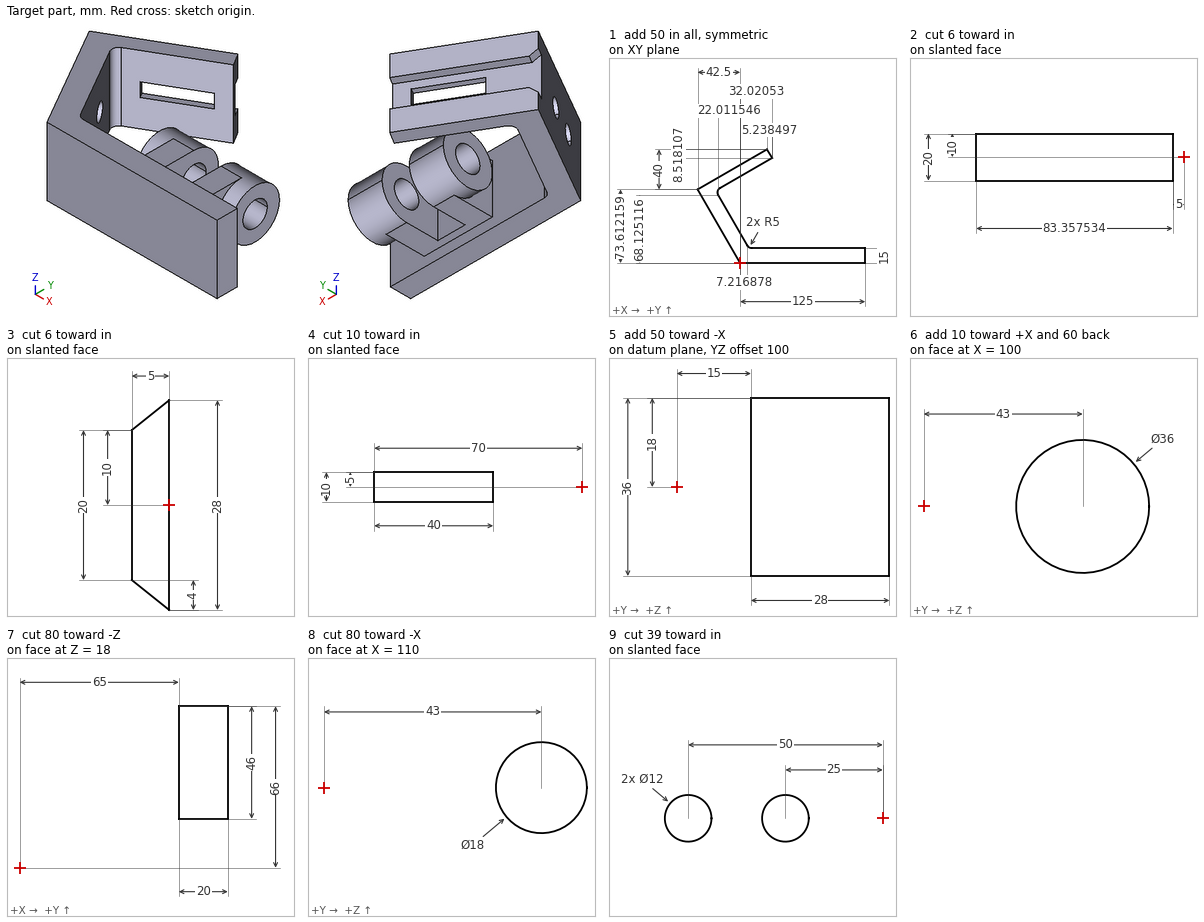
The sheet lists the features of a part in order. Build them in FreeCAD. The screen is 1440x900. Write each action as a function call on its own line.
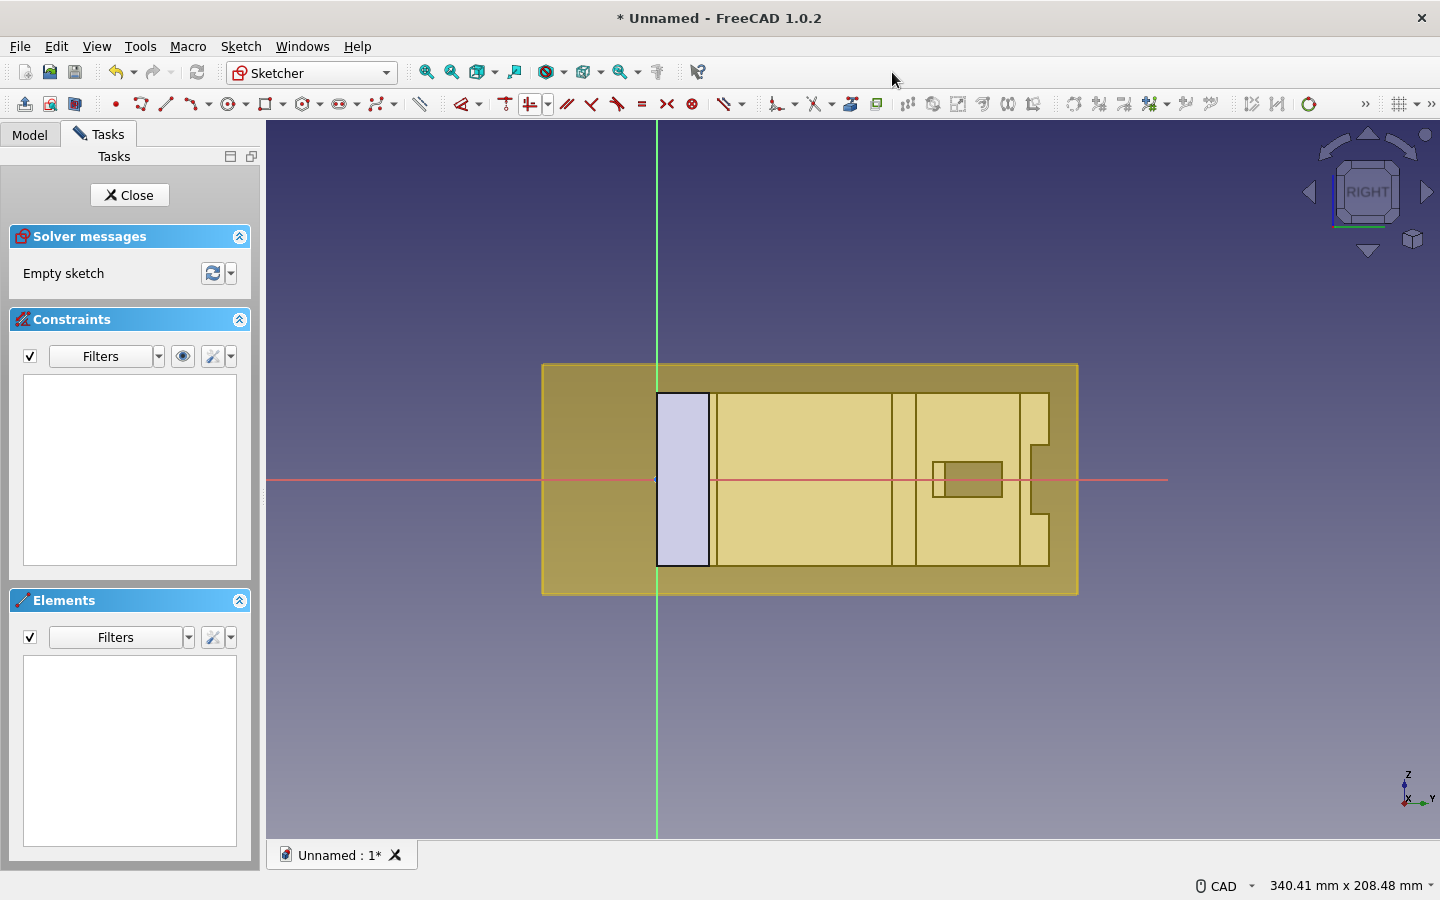
click(75, 104)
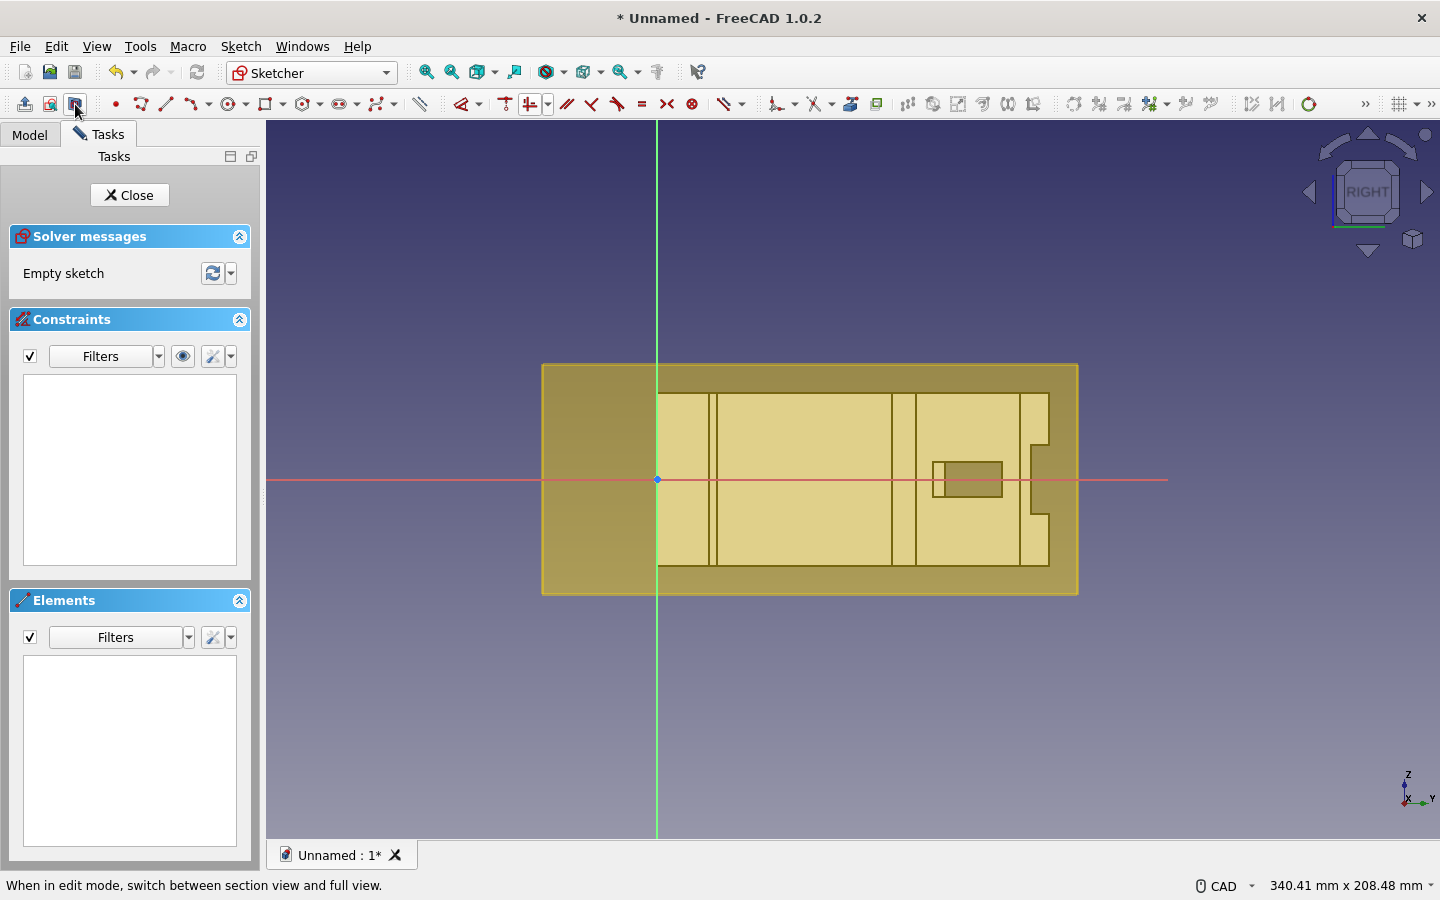
scroll(714, 480, up, 7)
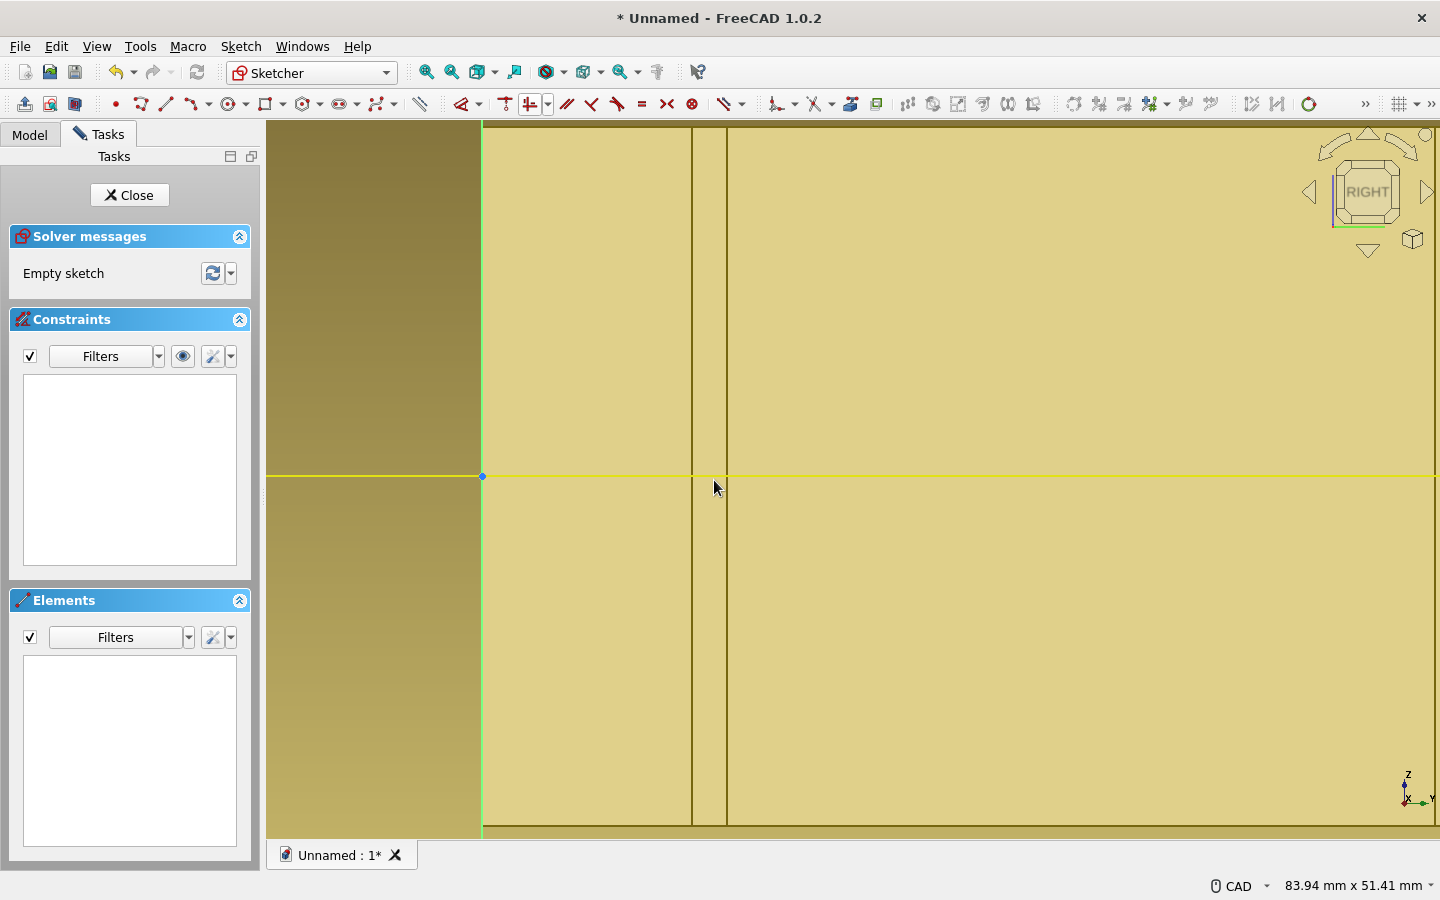
key(g)
key(r)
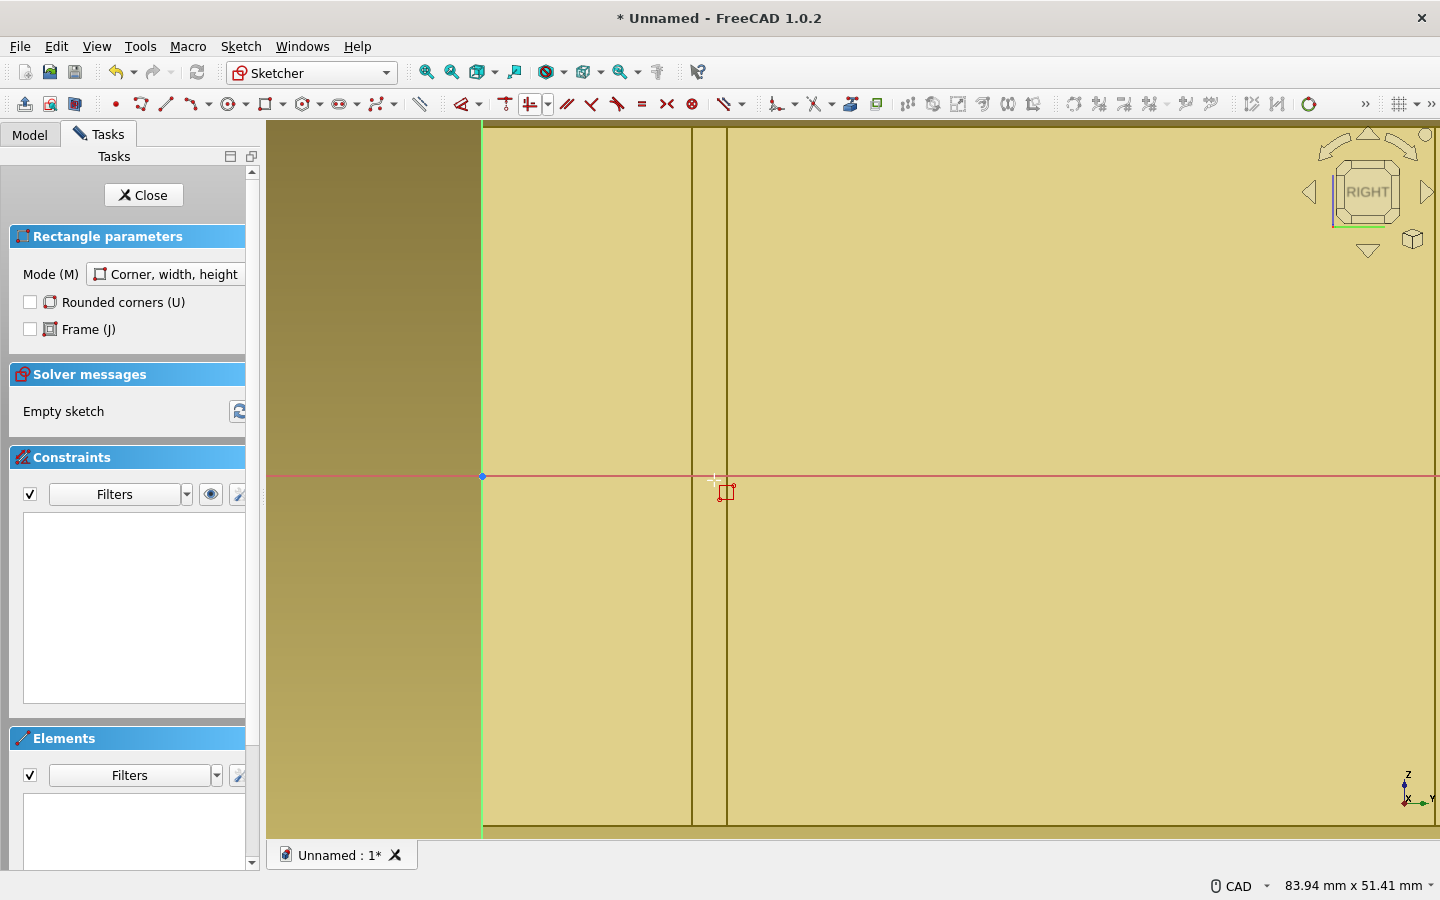
click(692, 225)
click(1083, 728)
key(Escape)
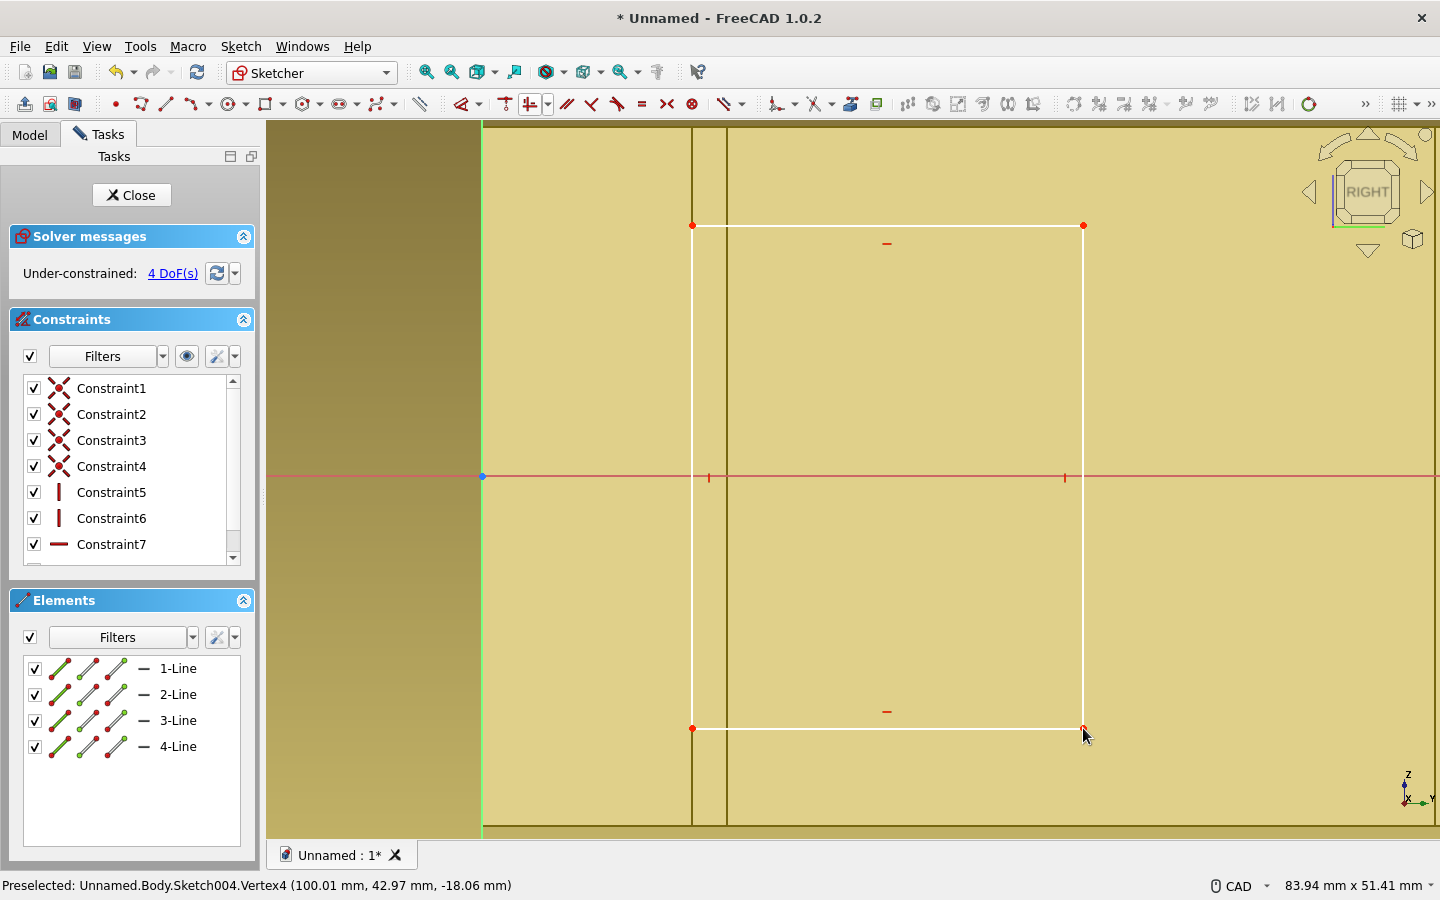
key(d)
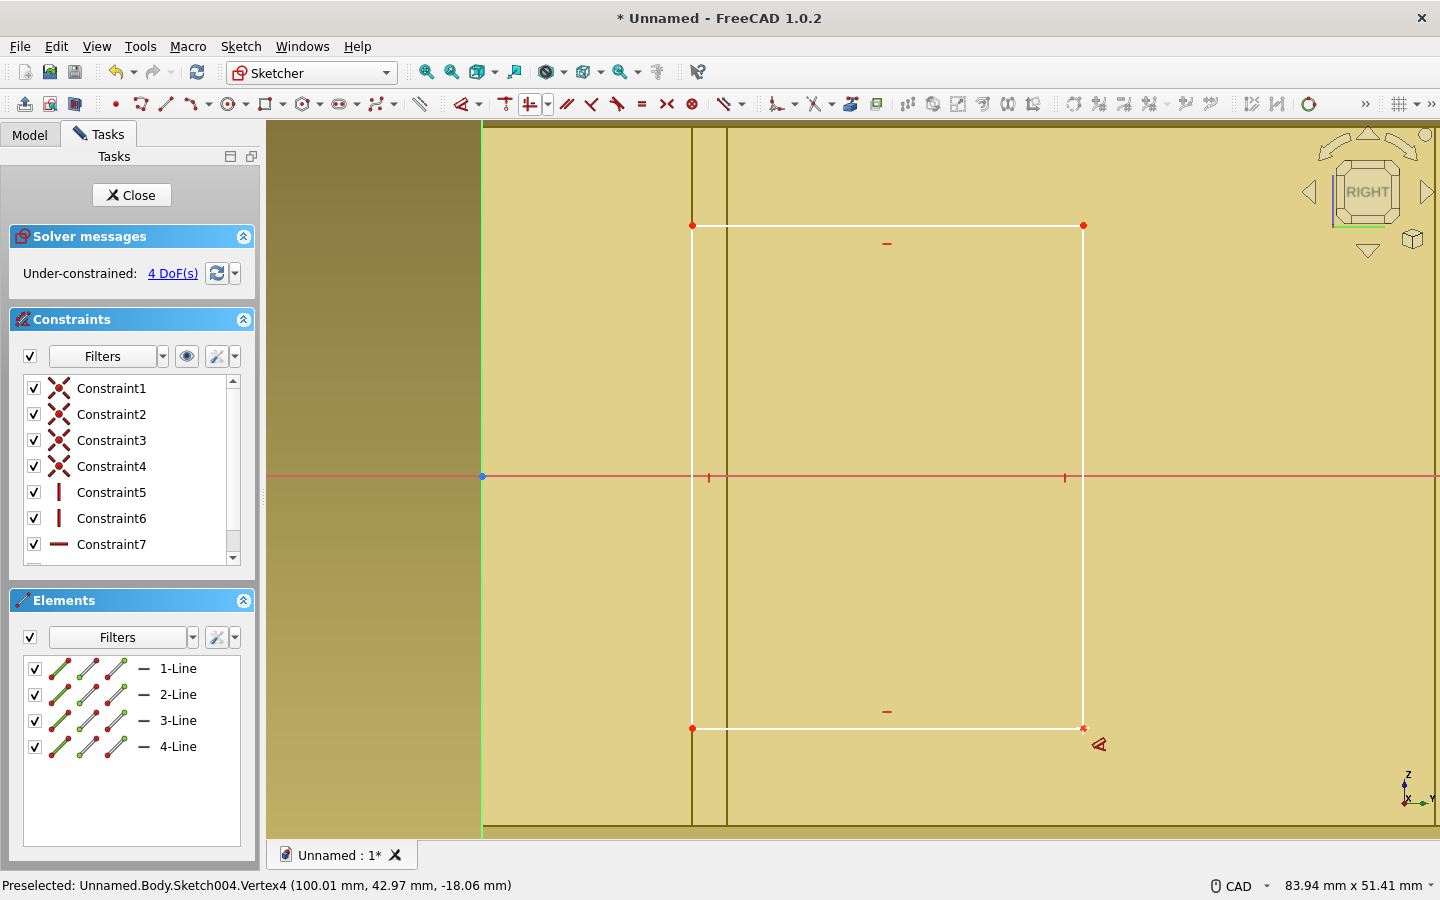
click(692, 377)
click(658, 362)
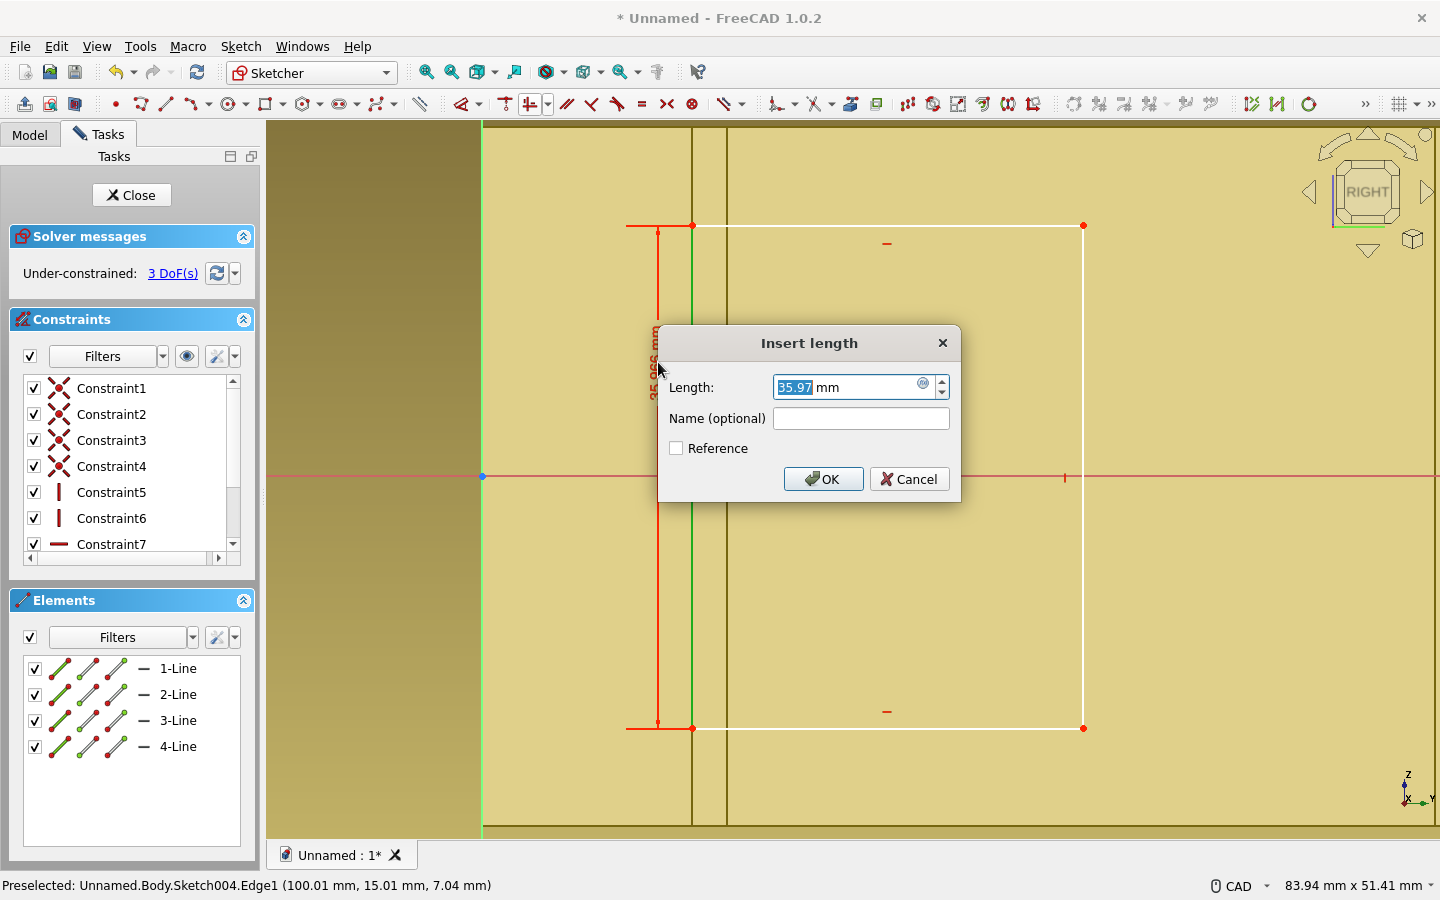
text(36)
key(Return)